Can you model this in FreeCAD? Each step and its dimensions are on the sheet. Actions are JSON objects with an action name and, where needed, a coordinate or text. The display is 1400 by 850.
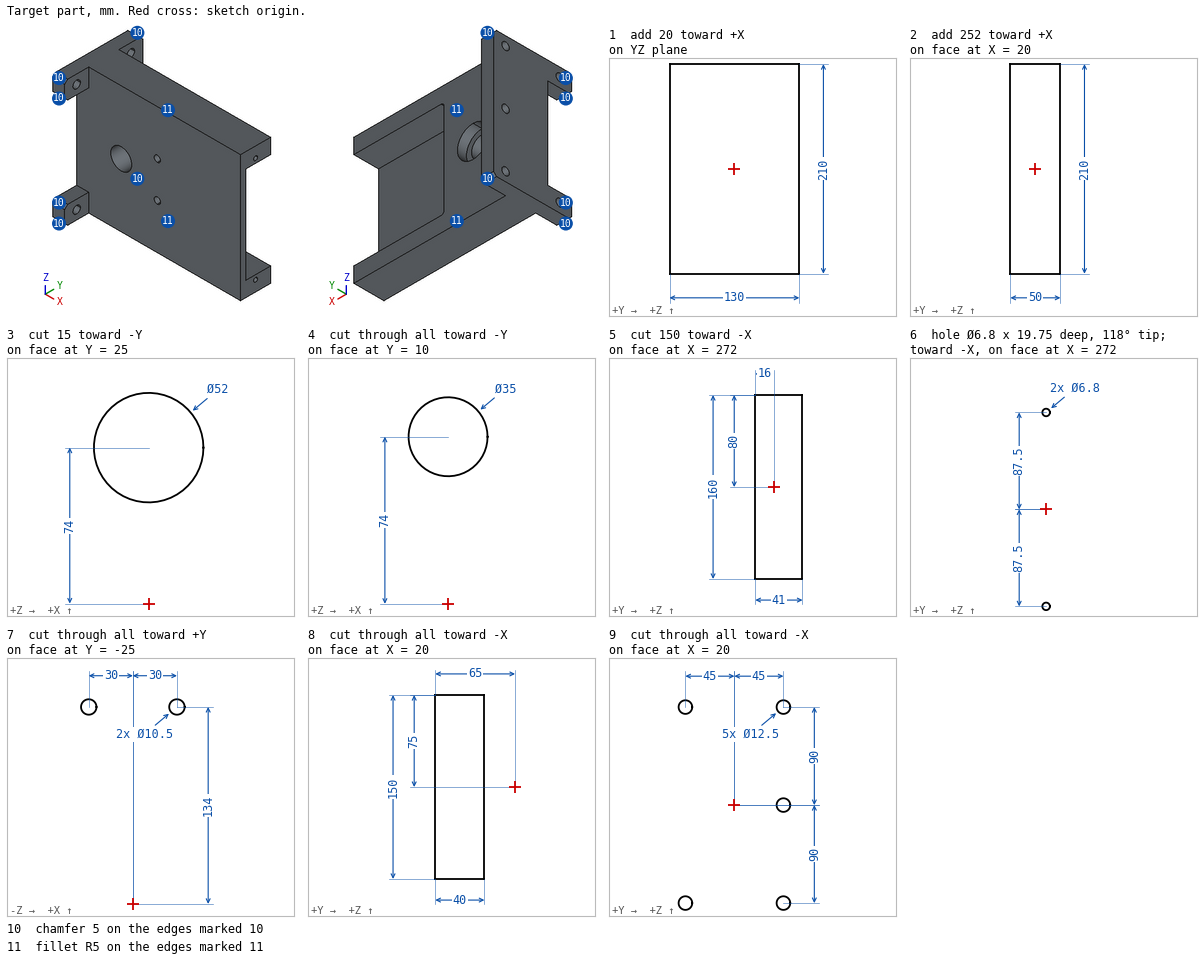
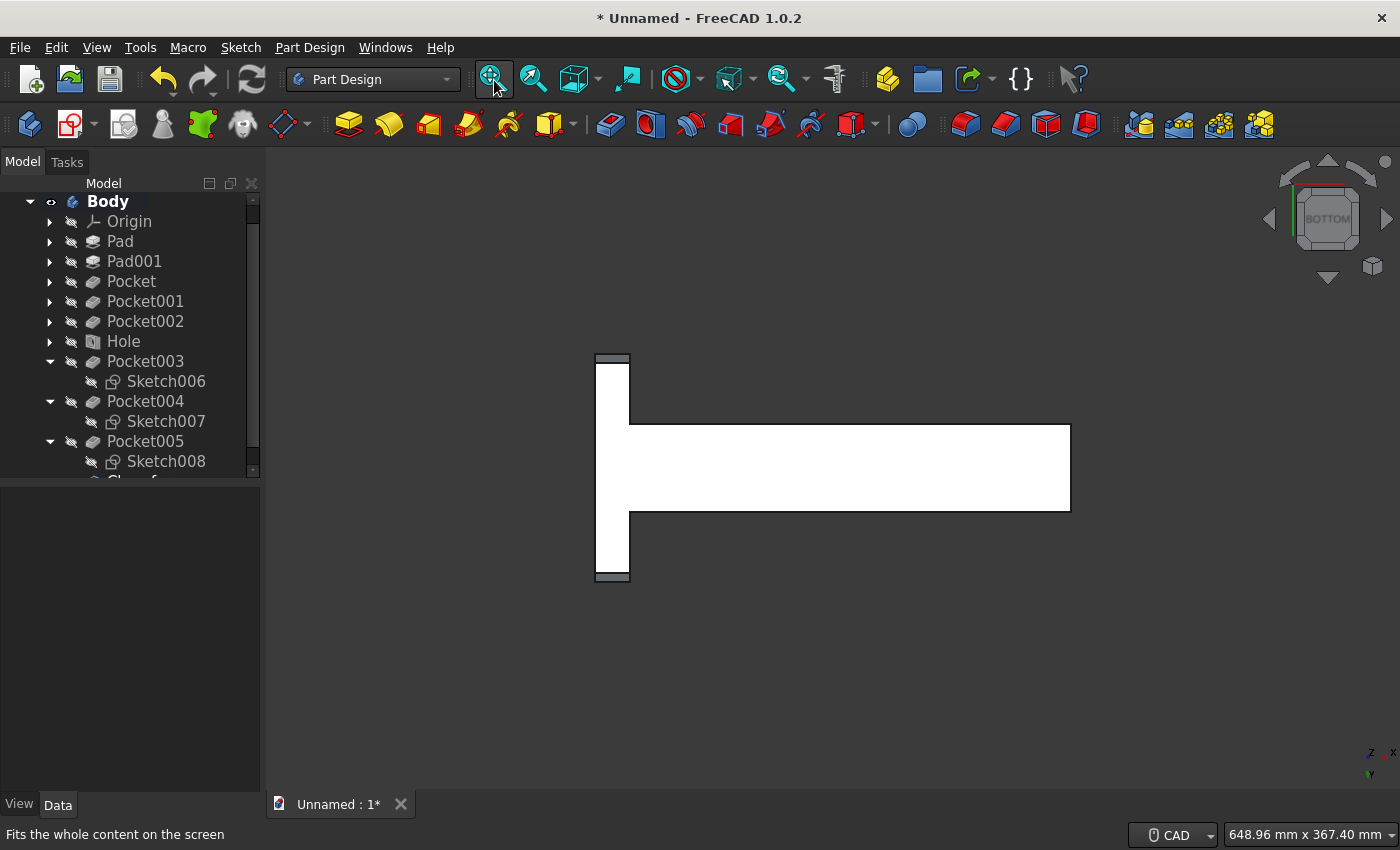
{"action": "key", "text": "0"}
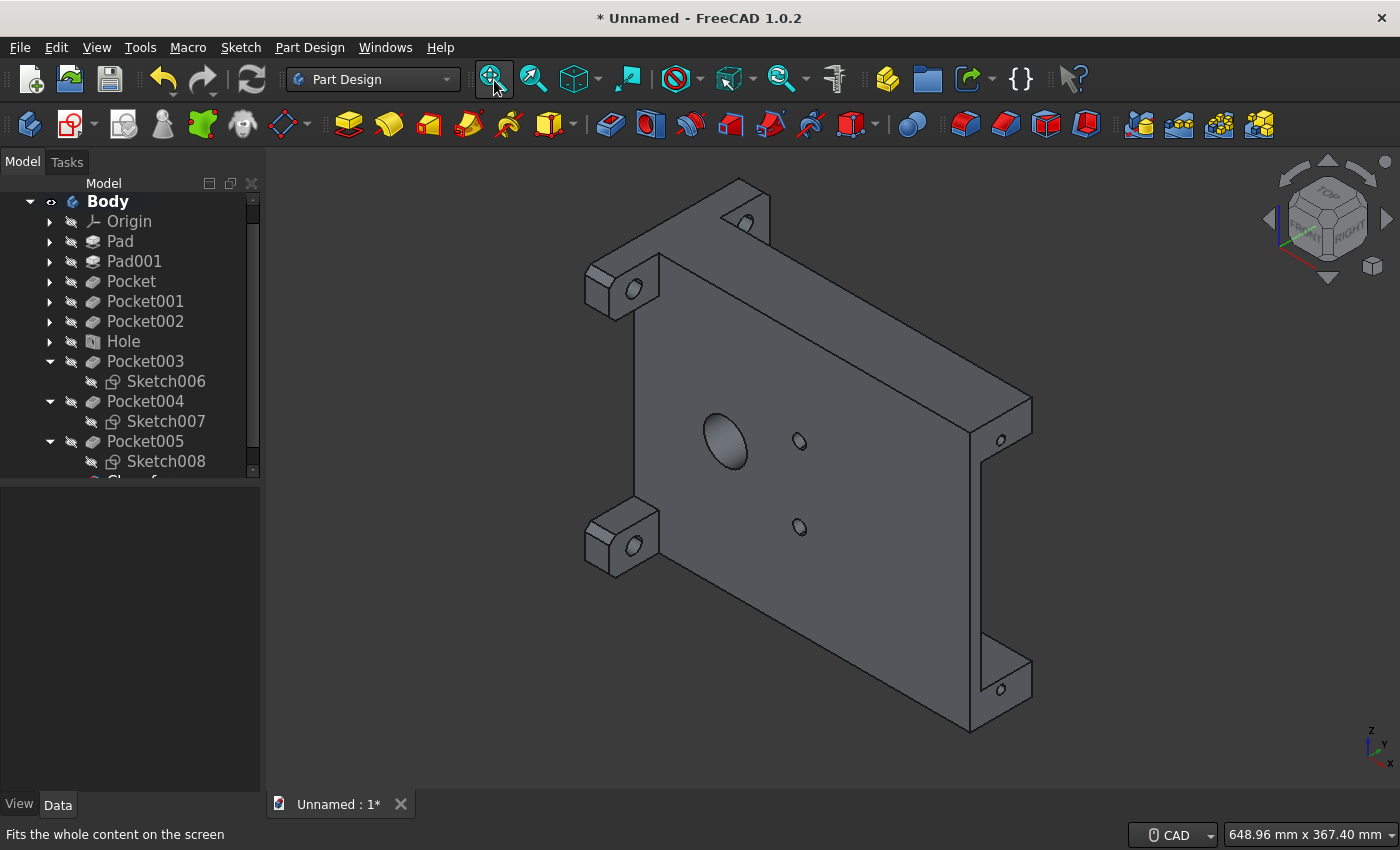
{"action": "key", "text": "2"}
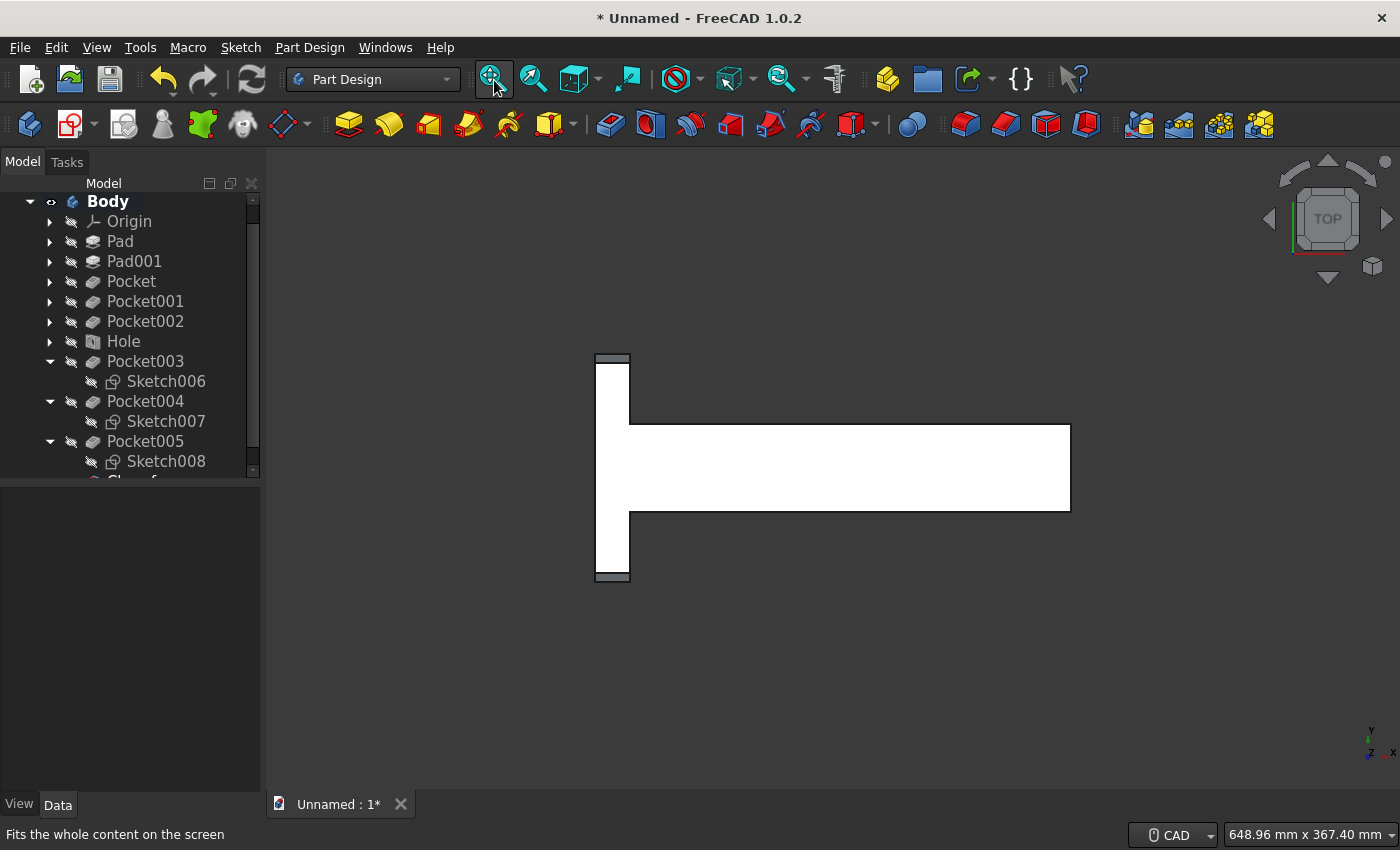
{"action": "left_click", "coordinate": [494, 80]}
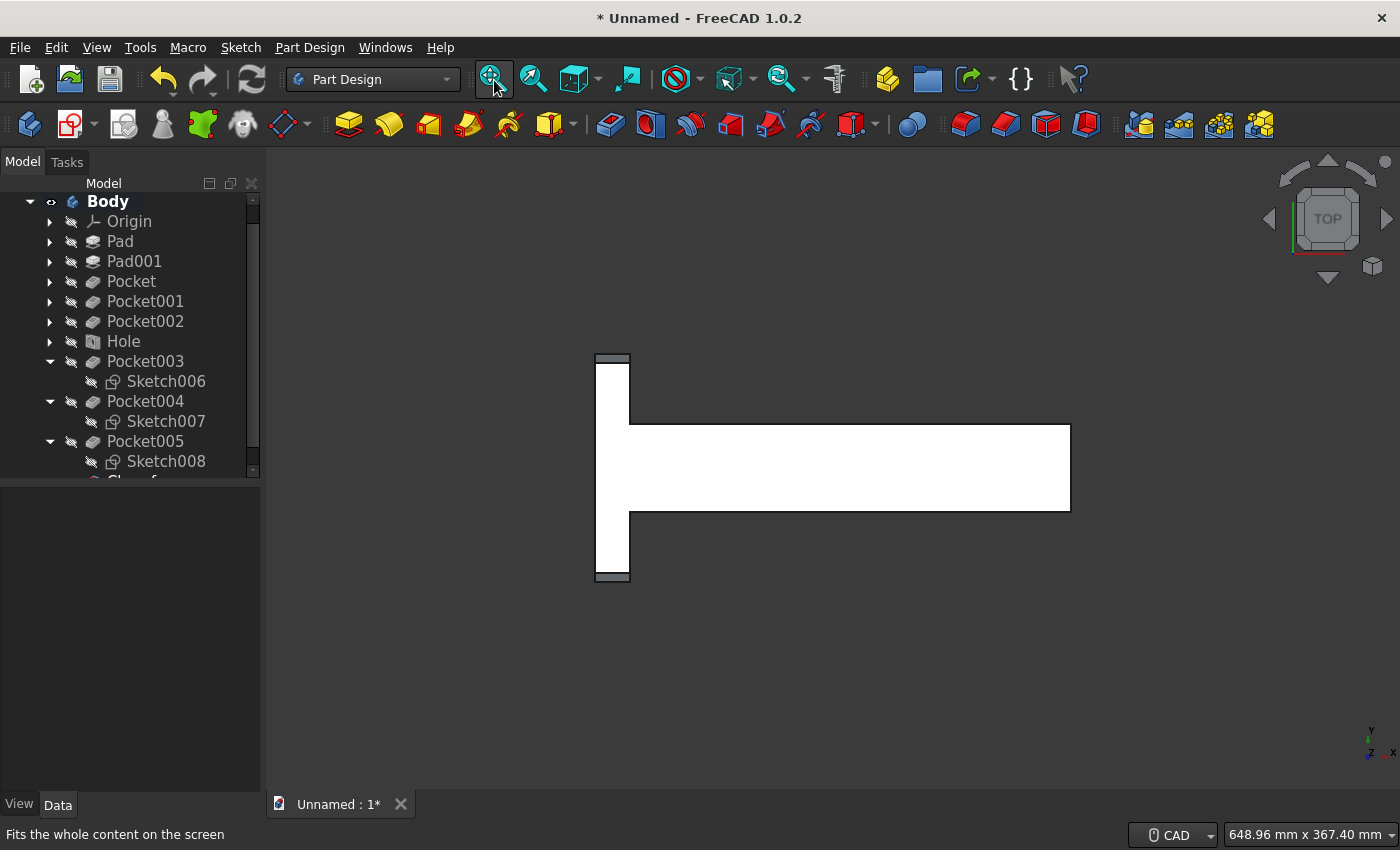
{"action": "key", "text": "1"}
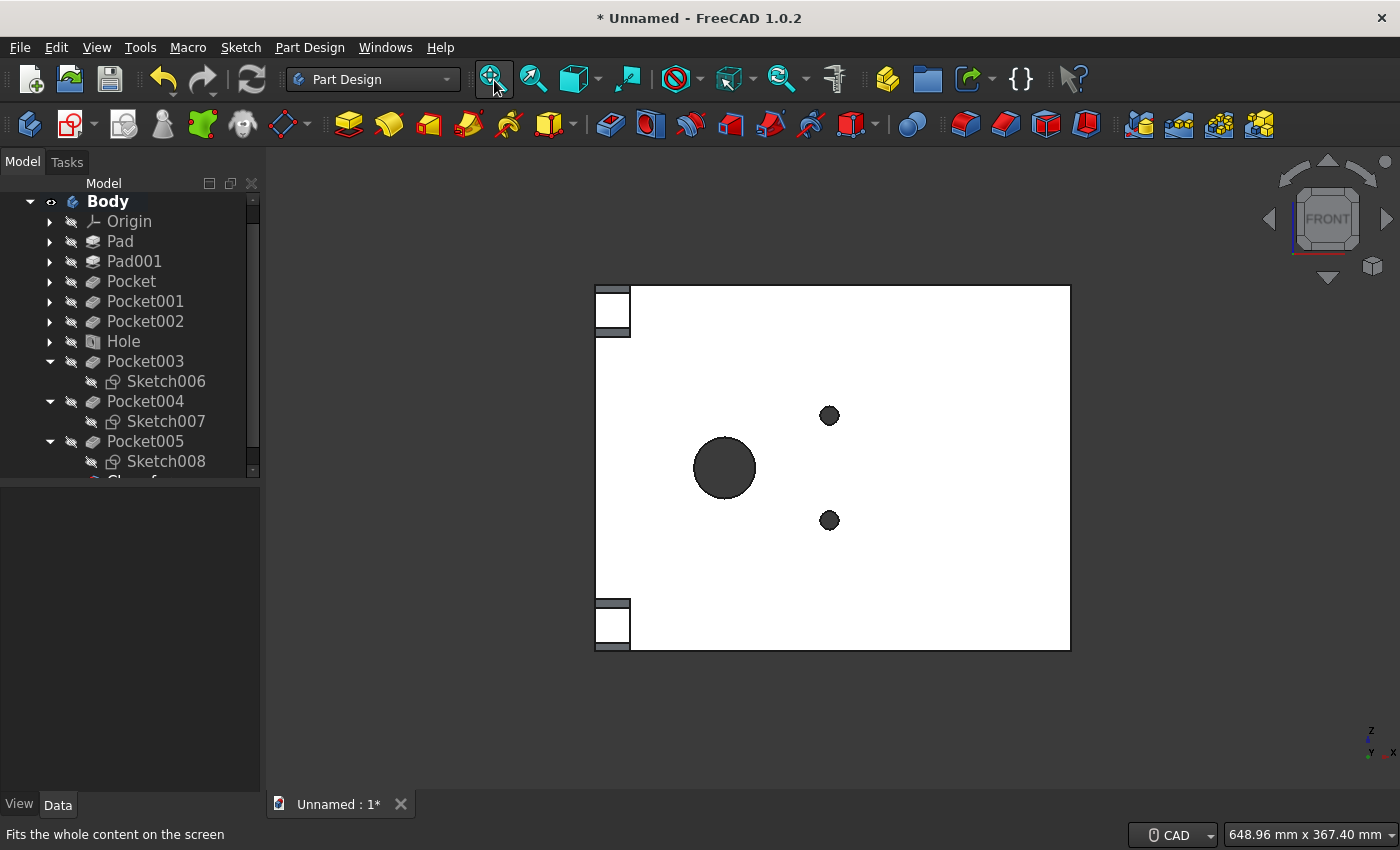
{"action": "key", "text": "3"}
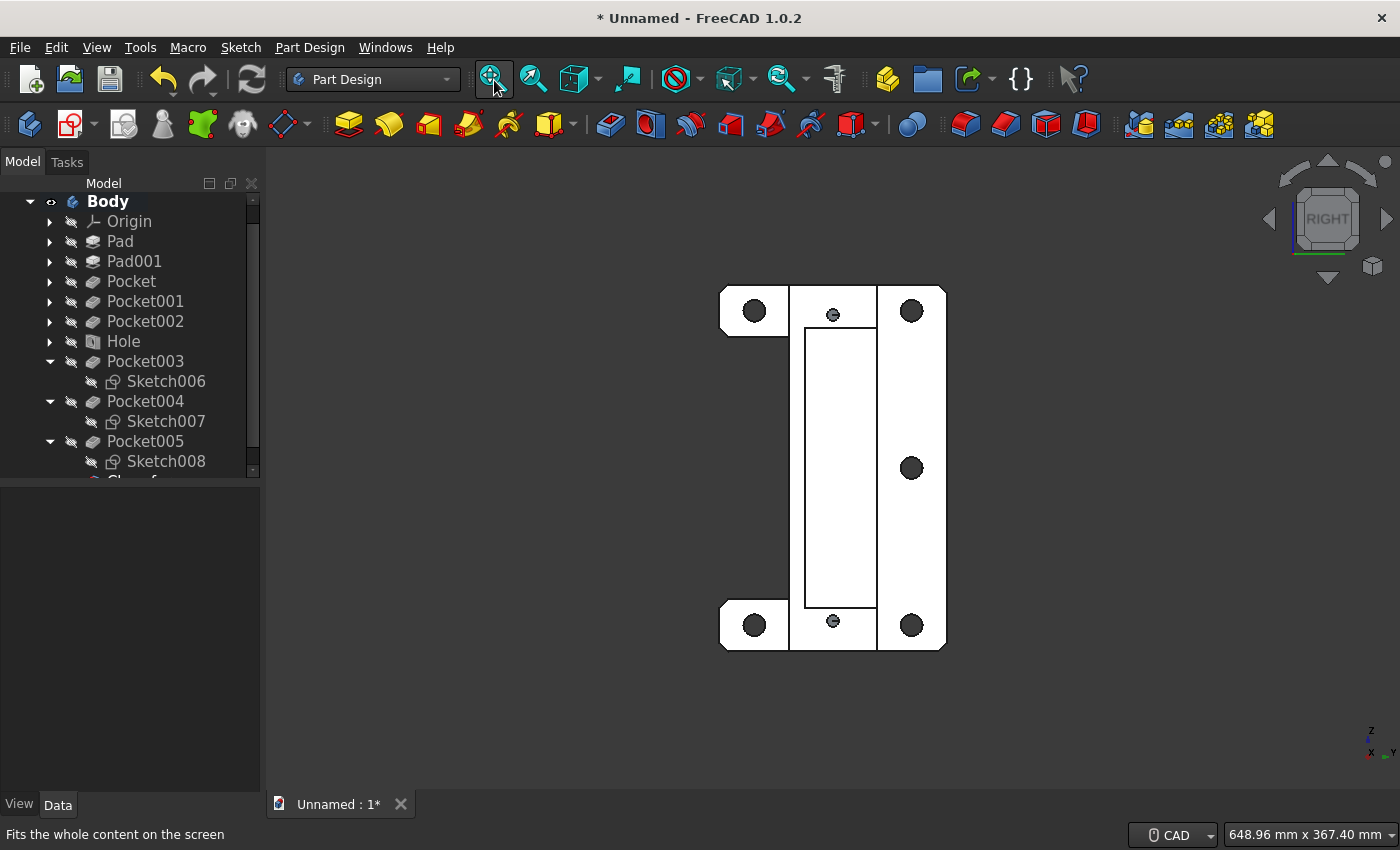
{"action": "key", "text": "5"}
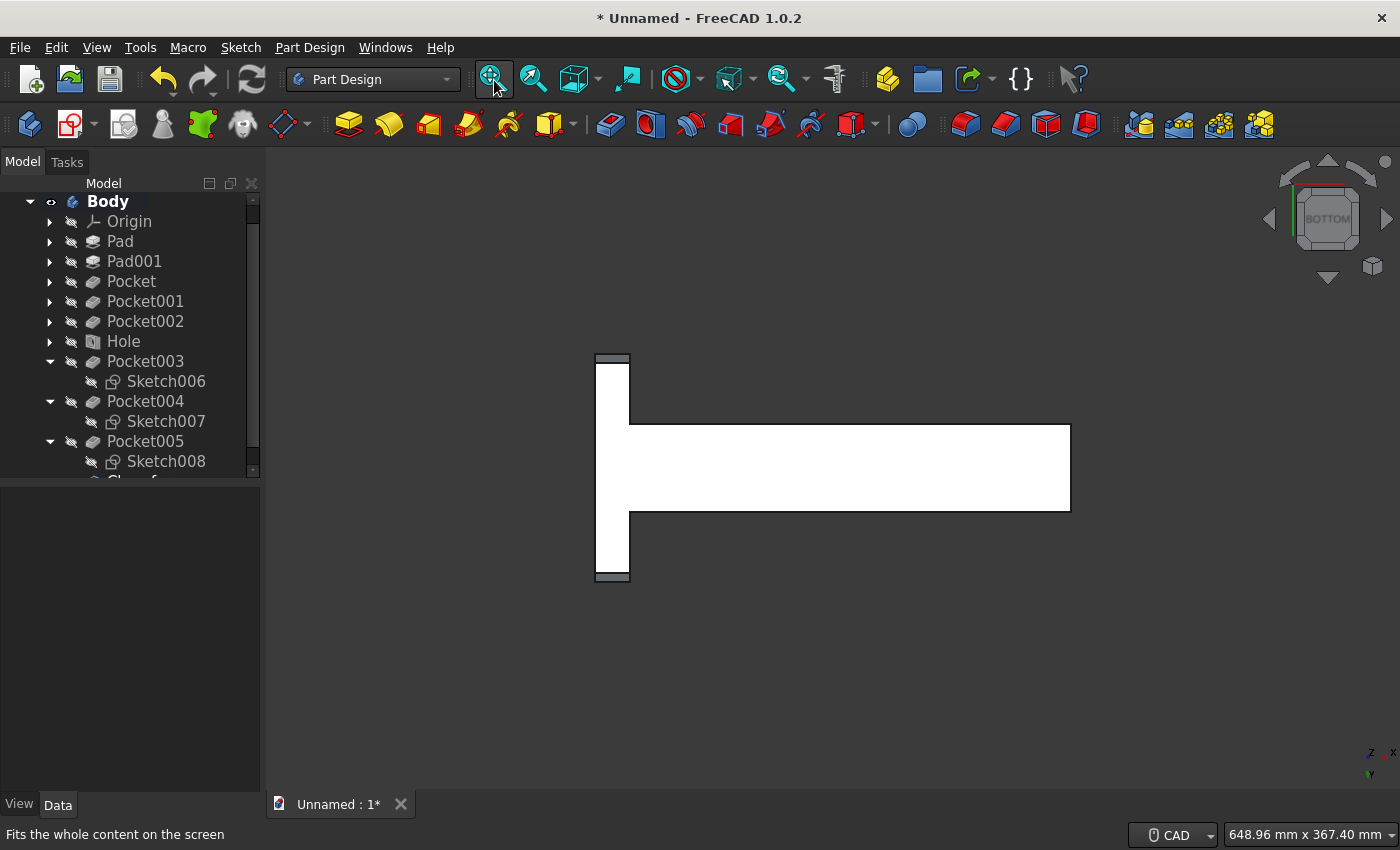
{"action": "left_click", "coordinate": [494, 80]}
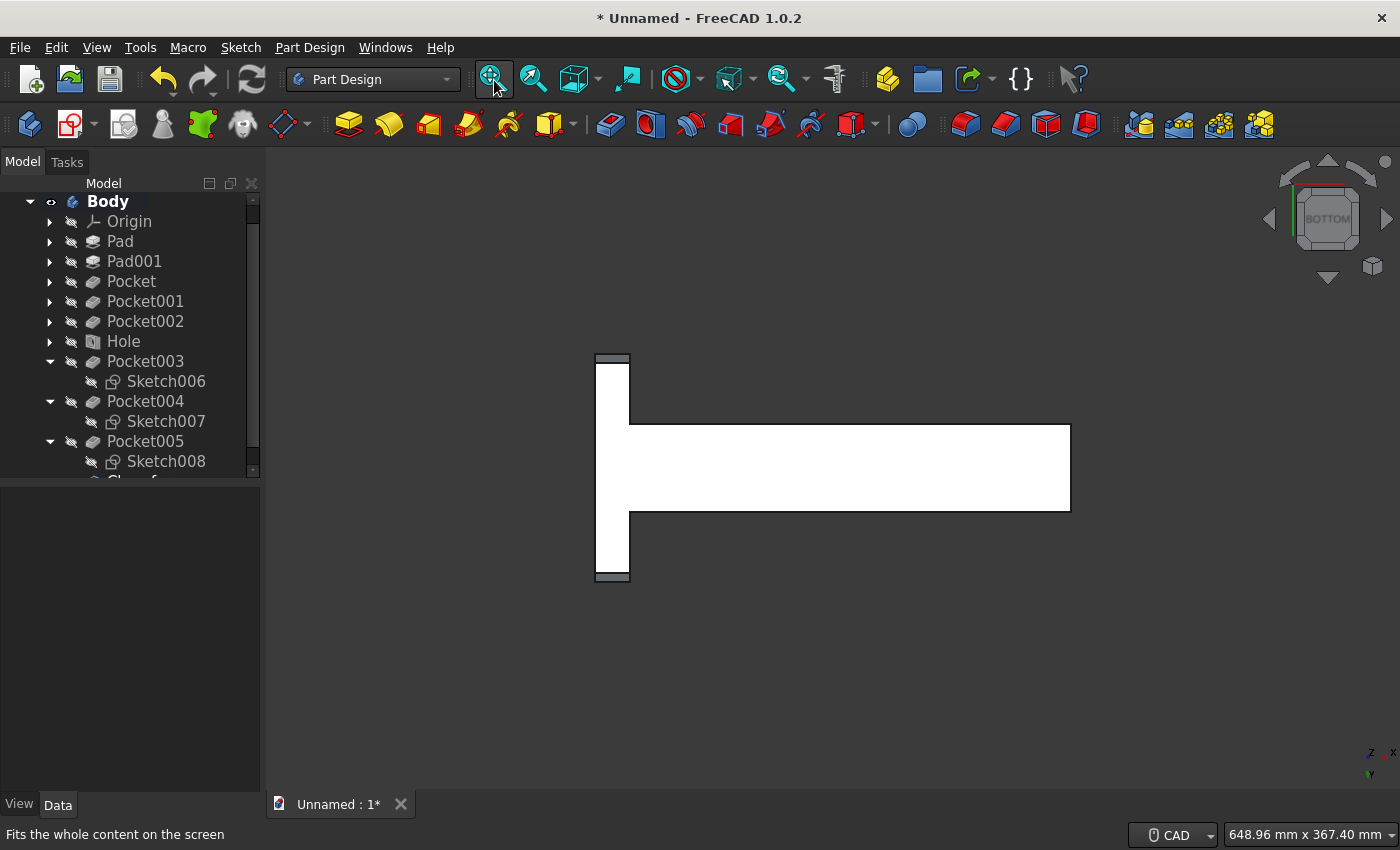
{"action": "key", "text": "4"}